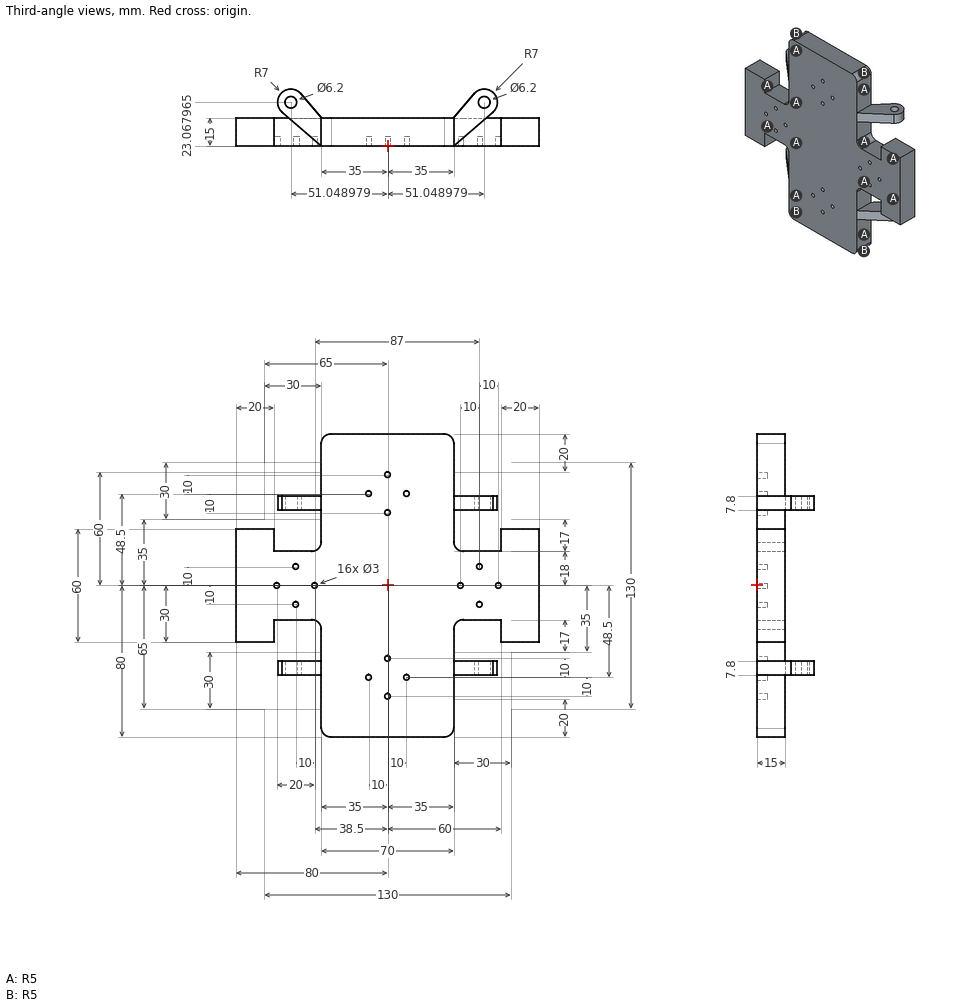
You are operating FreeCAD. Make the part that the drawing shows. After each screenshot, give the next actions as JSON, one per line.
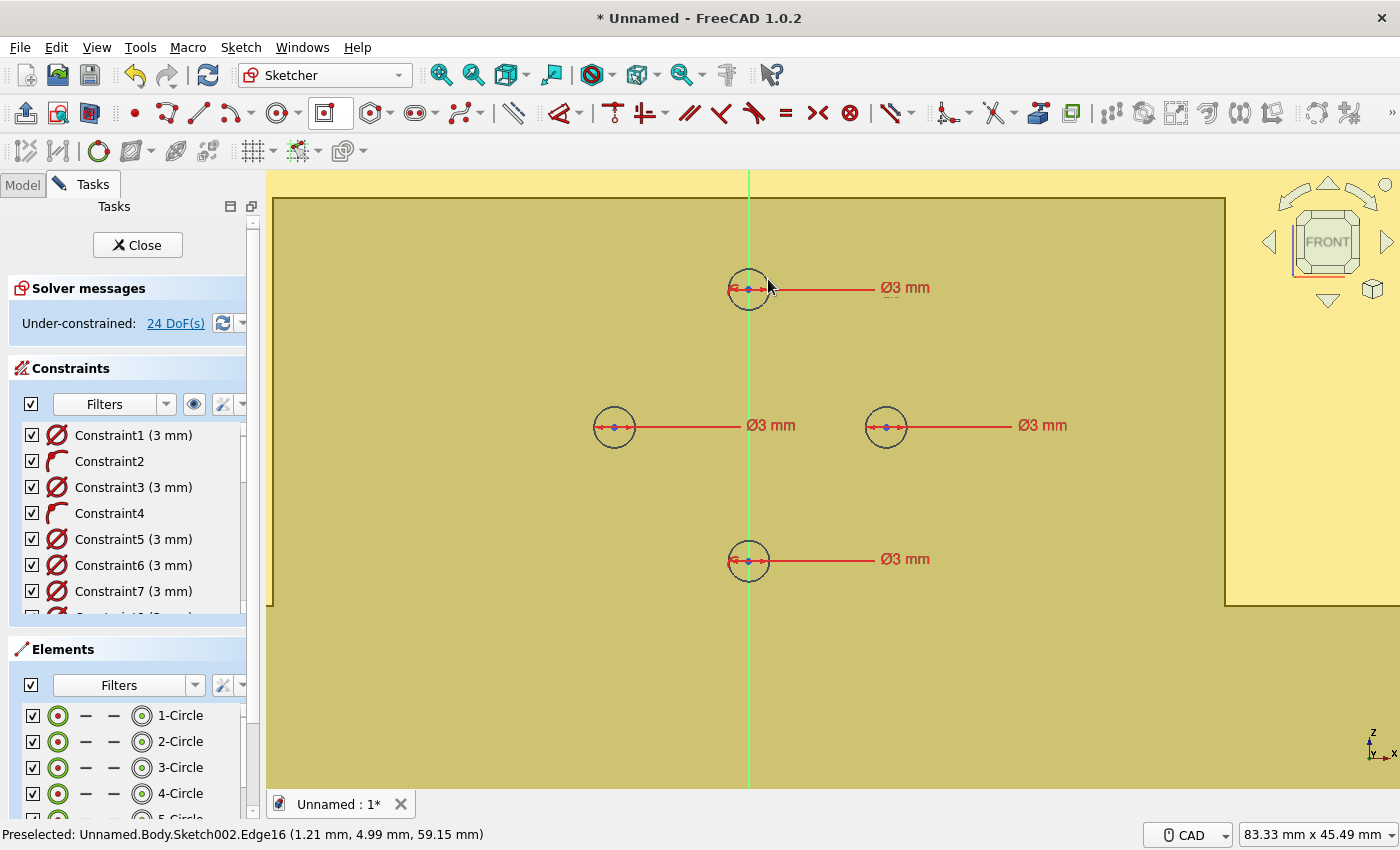
{"action": "left_click", "coordinate": [560, 114]}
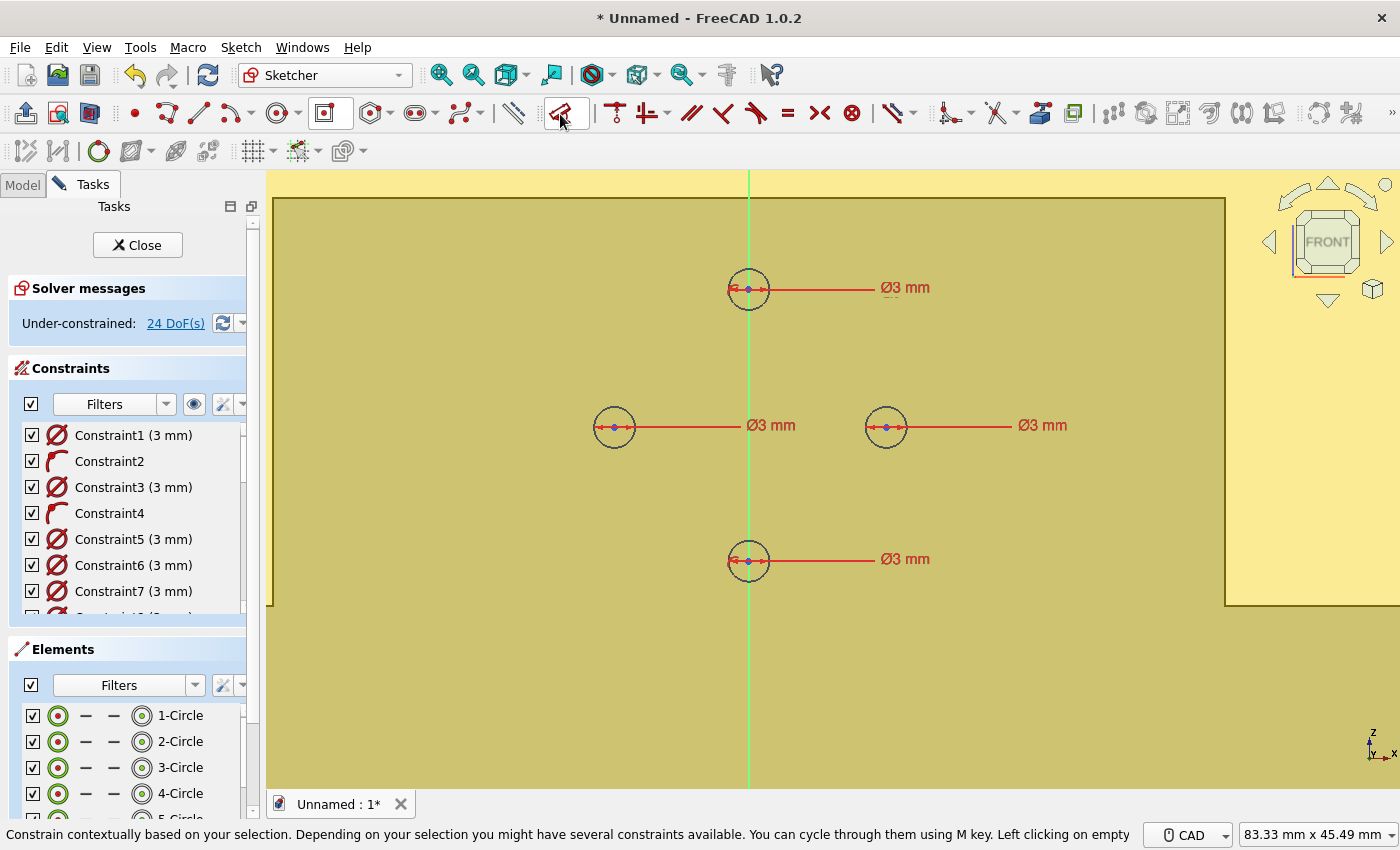
{"action": "scroll", "coordinate": [770, 282], "scroll_direction": "down", "scroll_amount": 7}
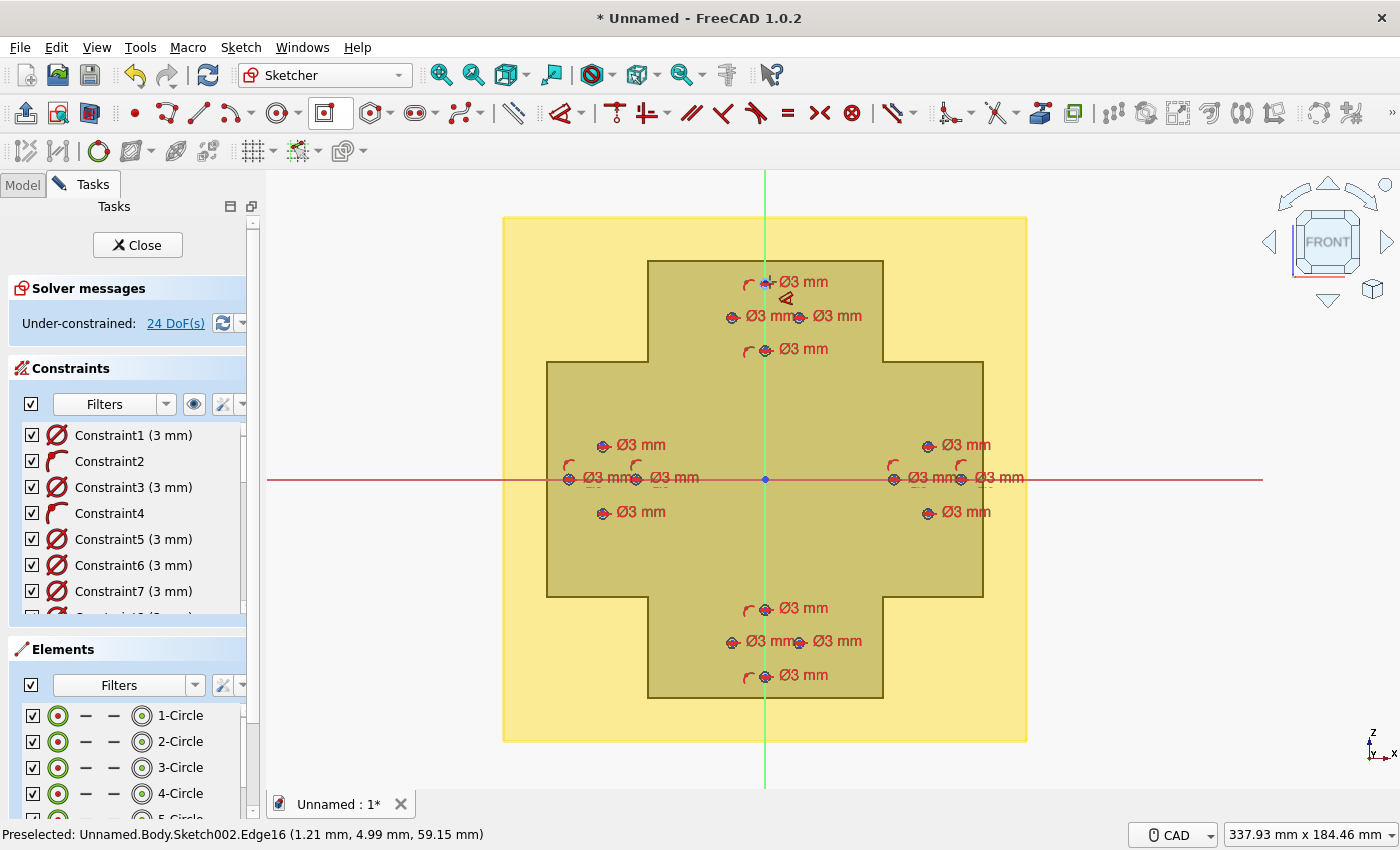
{"action": "left_click", "coordinate": [603, 514]}
{"action": "left_click", "coordinate": [569, 505]}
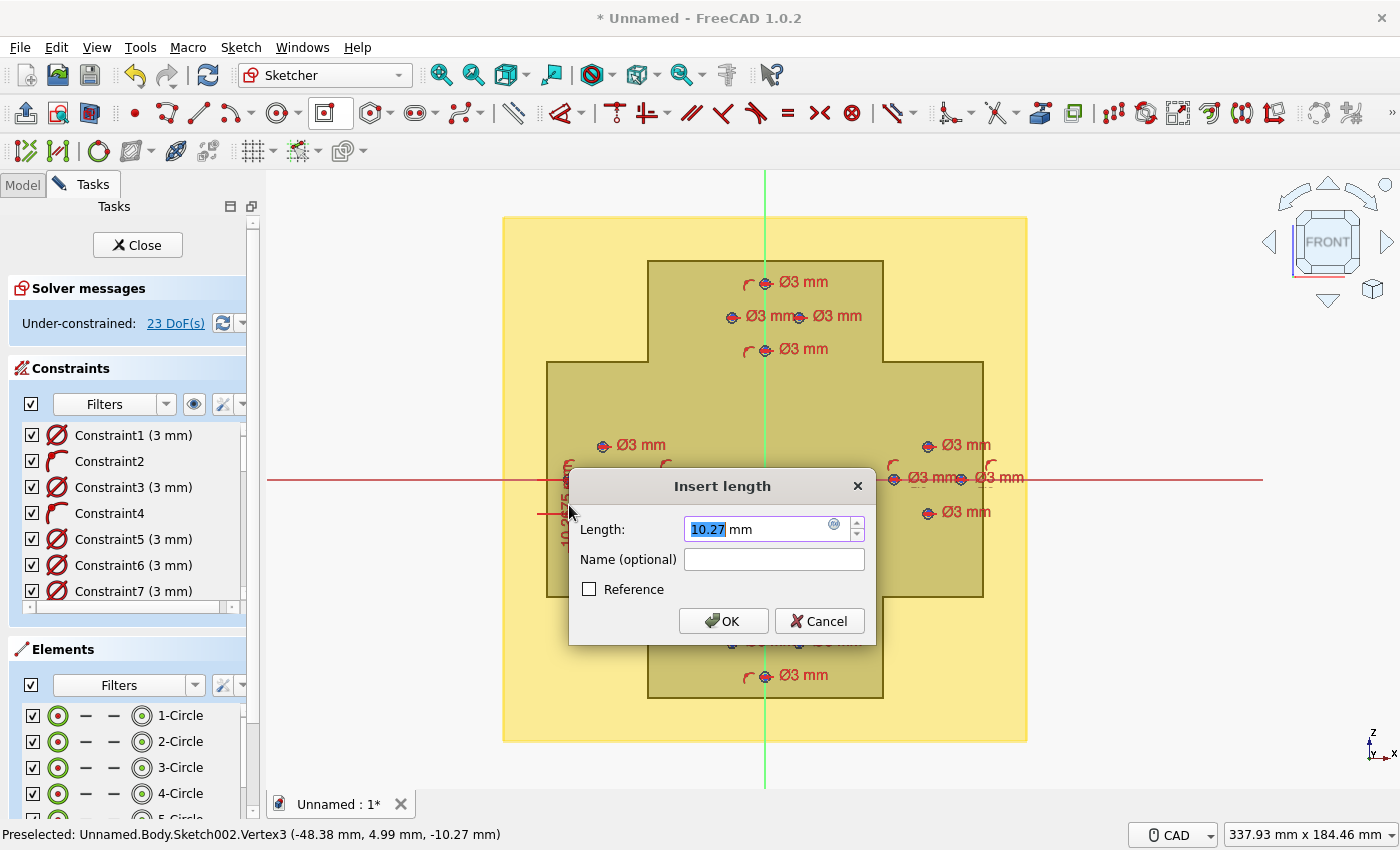
{"action": "type", "text": "10"}
{"action": "key", "text": "Return"}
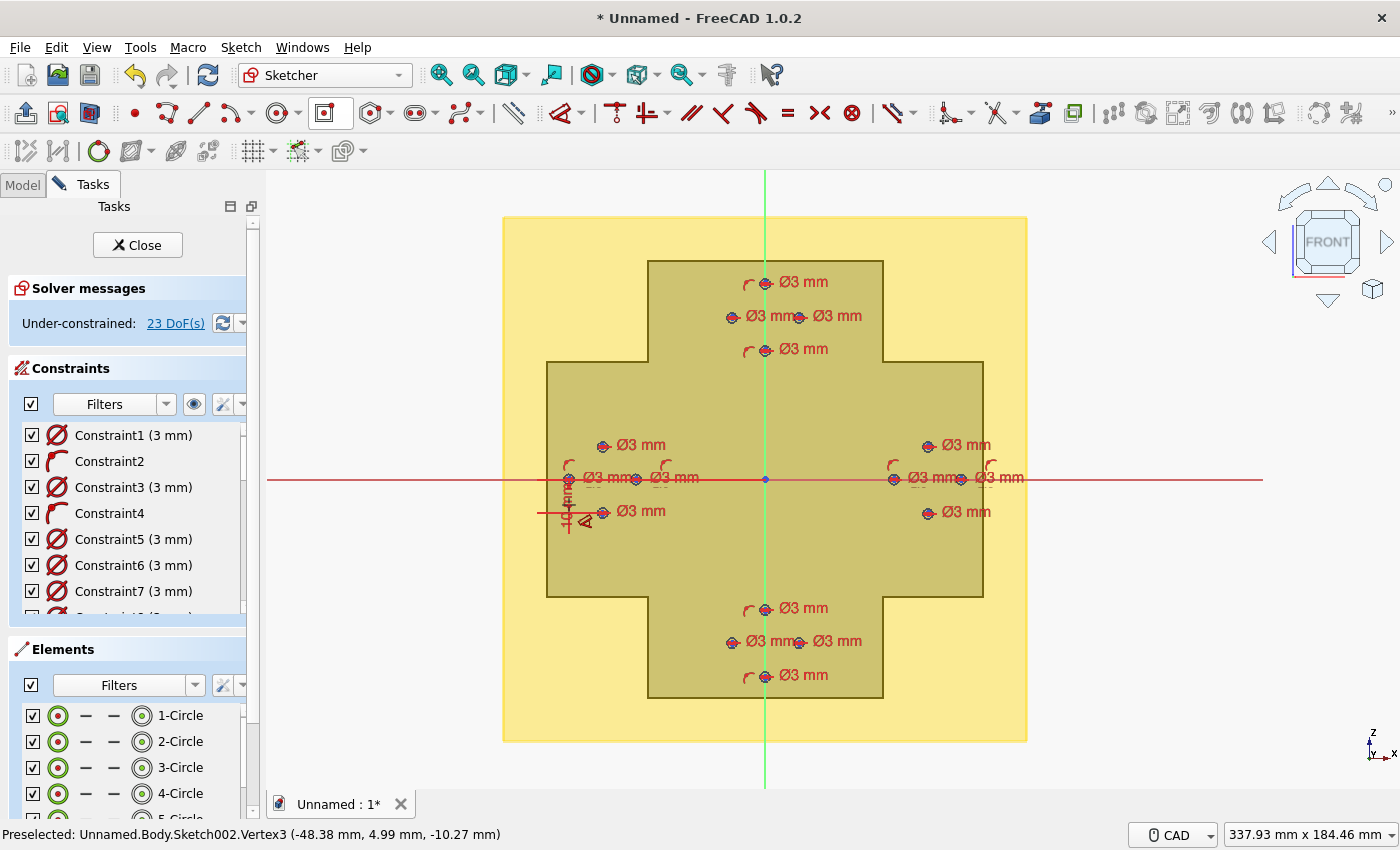
{"action": "left_click", "coordinate": [603, 447]}
{"action": "left_click", "coordinate": [569, 456]}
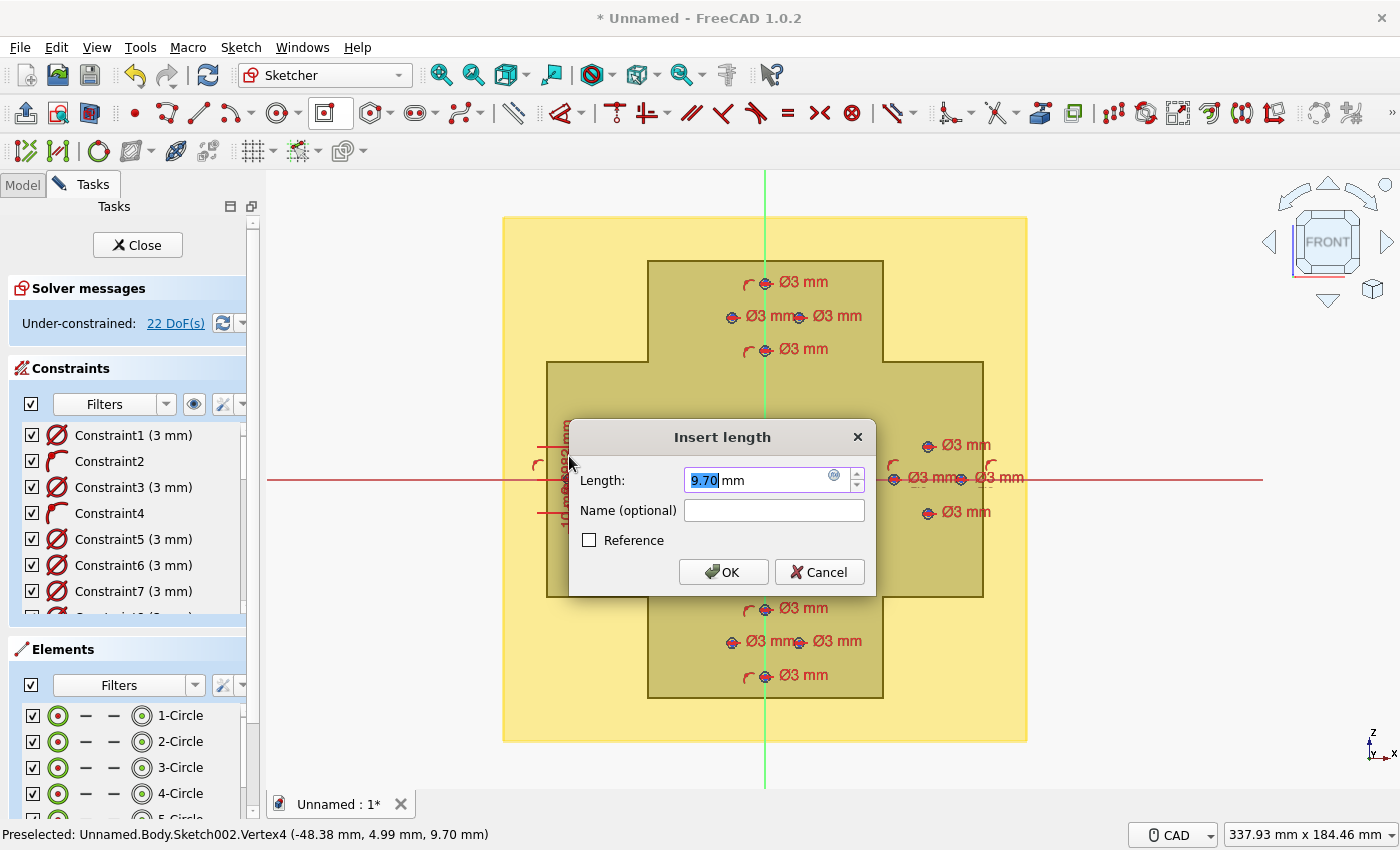
{"action": "type", "text": "10"}
{"action": "key", "text": "Return"}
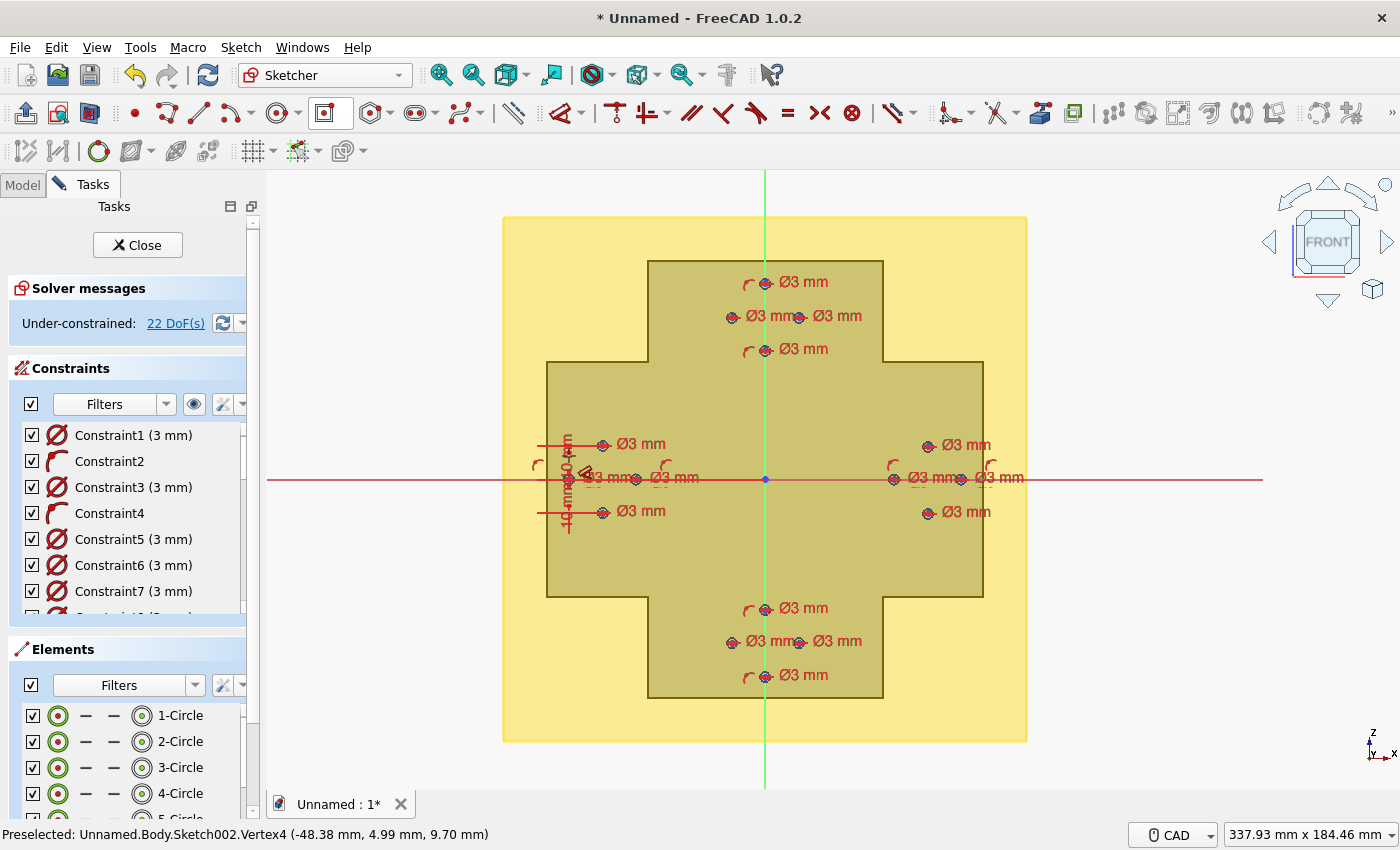
{"action": "left_click", "coordinate": [799, 643]}
{"action": "left_click", "coordinate": [790, 677]}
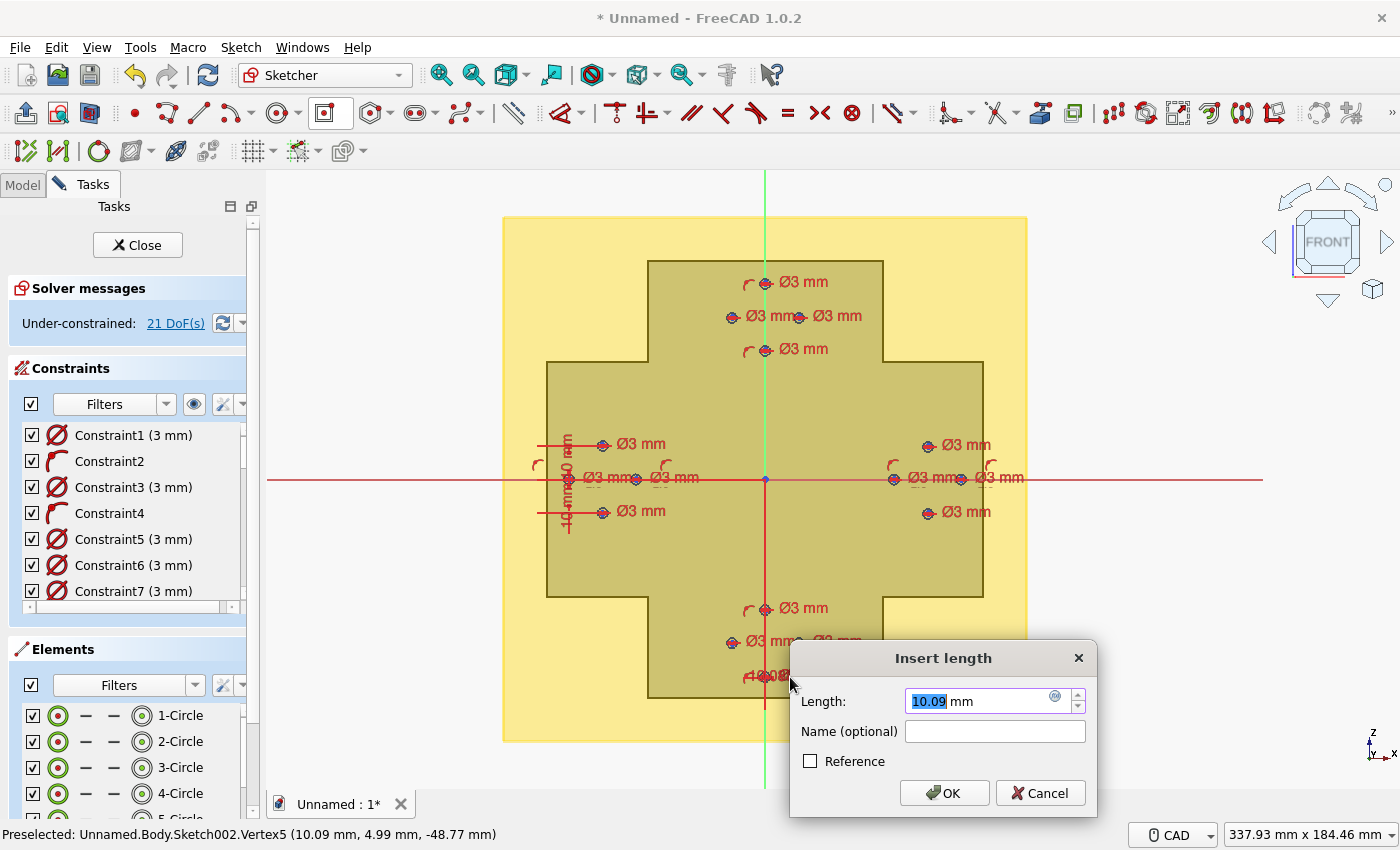
{"action": "type", "text": "10"}
{"action": "key", "text": "Return"}